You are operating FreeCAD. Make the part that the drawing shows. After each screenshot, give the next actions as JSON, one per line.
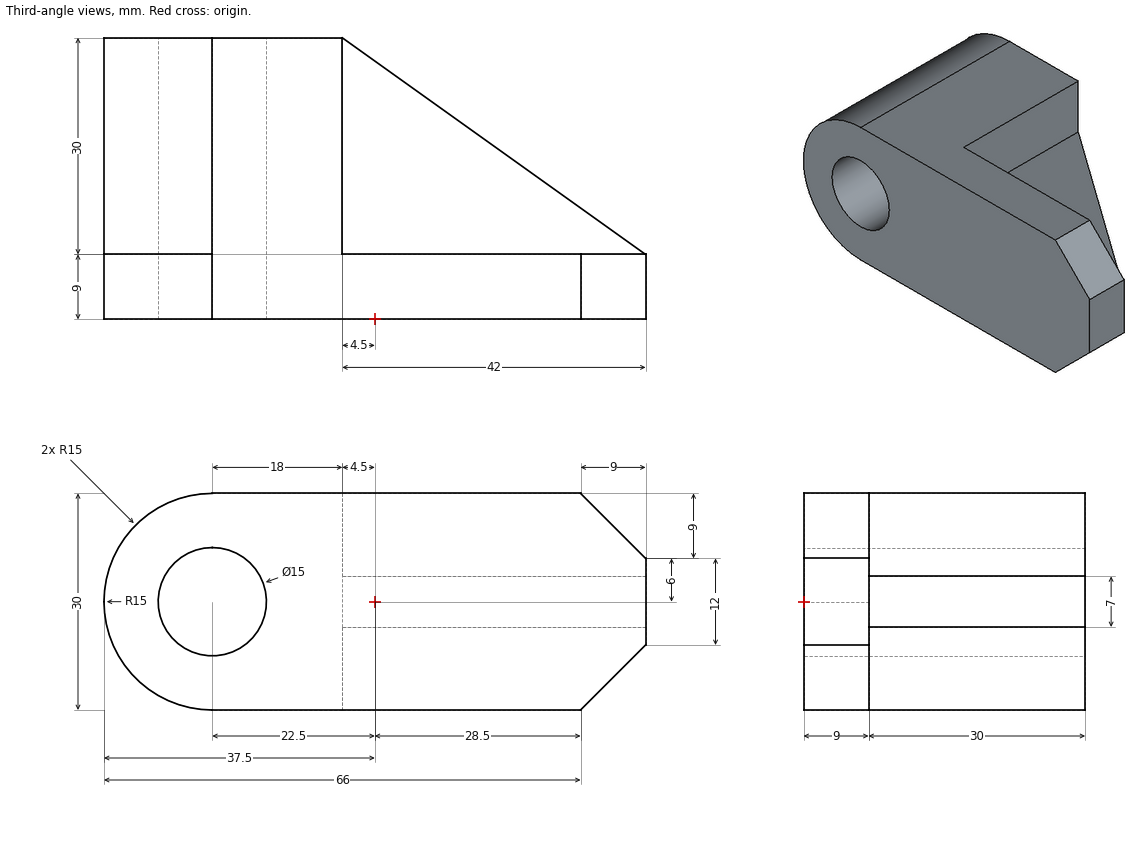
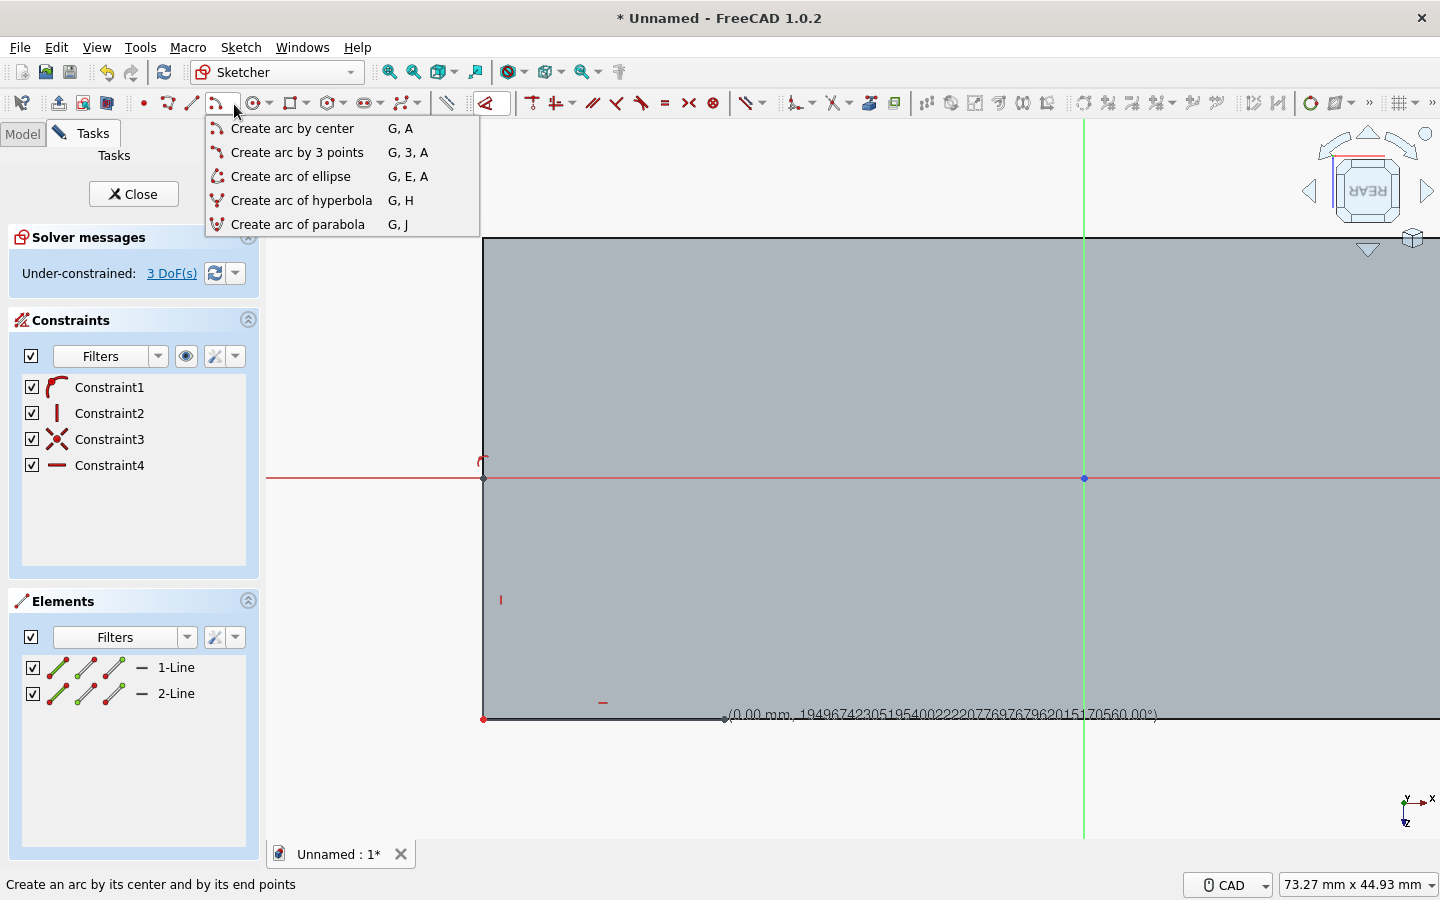
{"action": "left_click", "coordinate": [342, 152]}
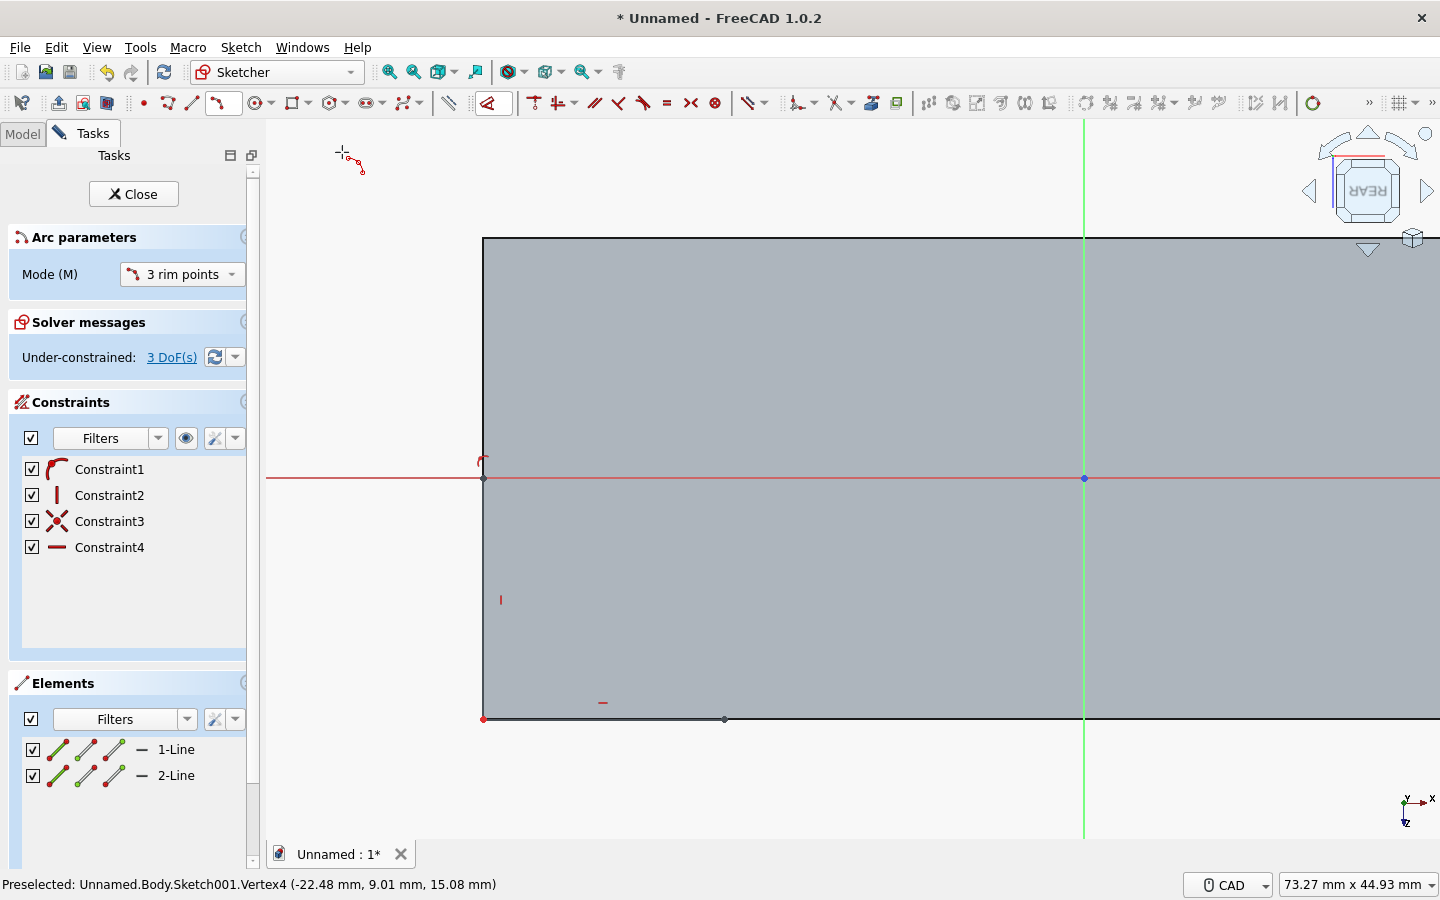
{"action": "left_click", "coordinate": [724, 720]}
{"action": "left_click", "coordinate": [483, 478]}
{"action": "left_click", "coordinate": [554, 648]}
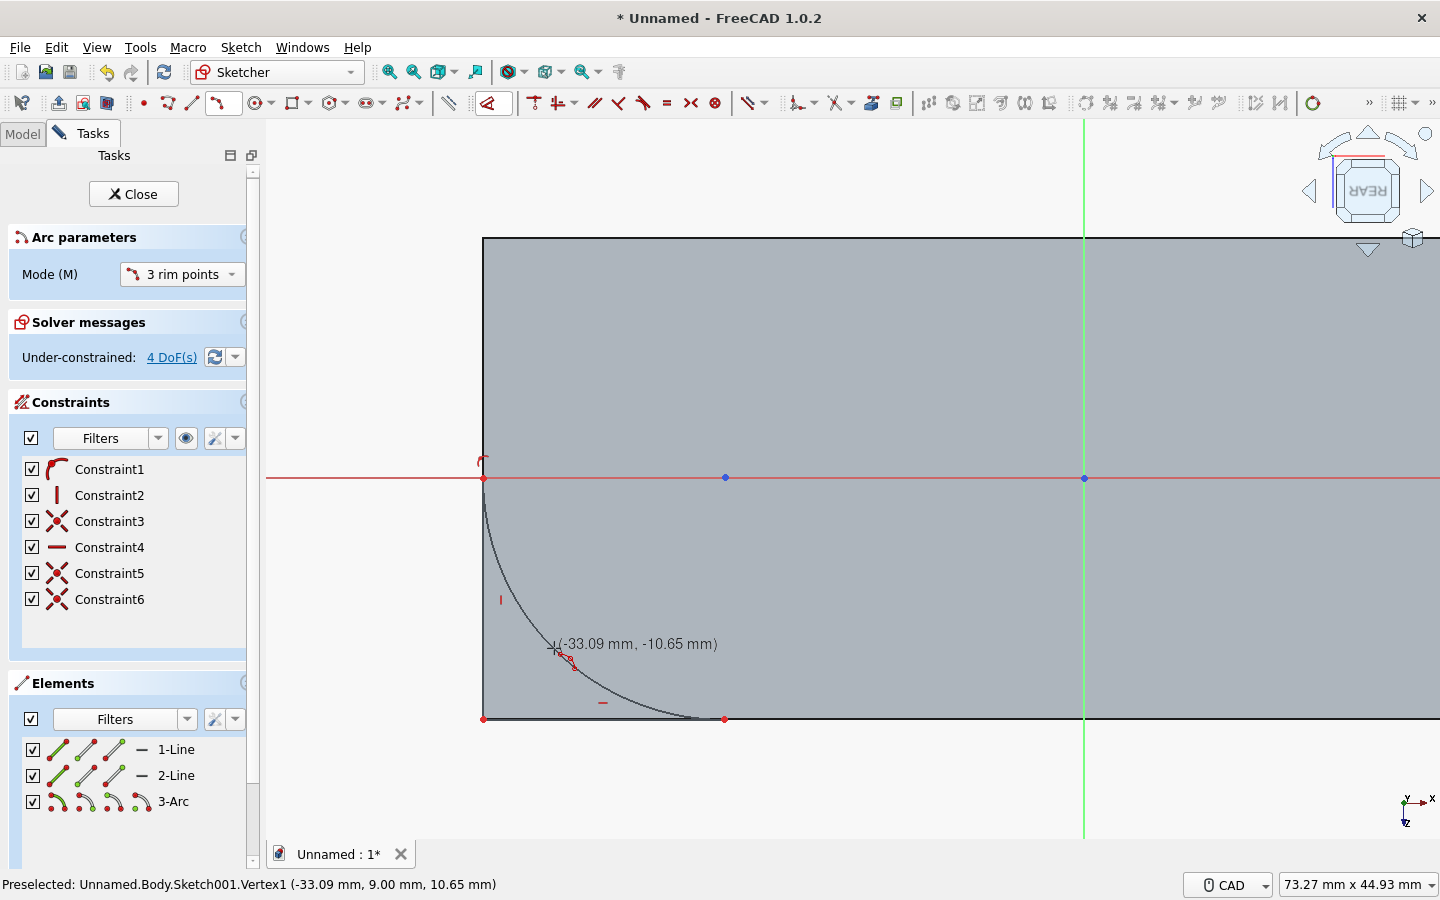
{"action": "key", "text": "g m"}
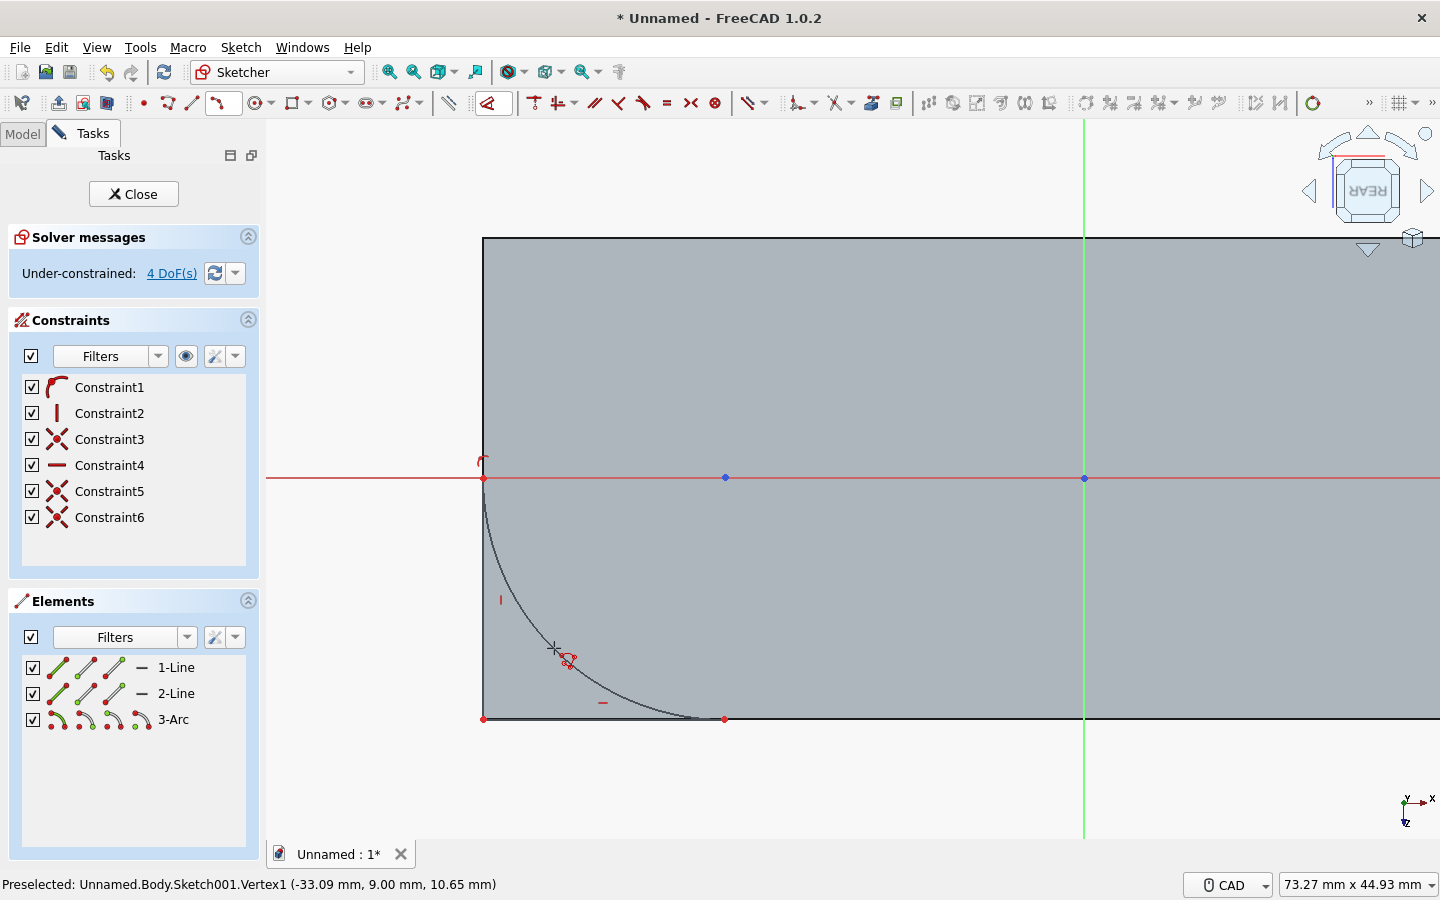
{"action": "left_click", "coordinate": [724, 238]}
{"action": "left_click", "coordinate": [483, 238]}
{"action": "left_click", "coordinate": [483, 478]}
{"action": "right_click", "coordinate": [483, 238]}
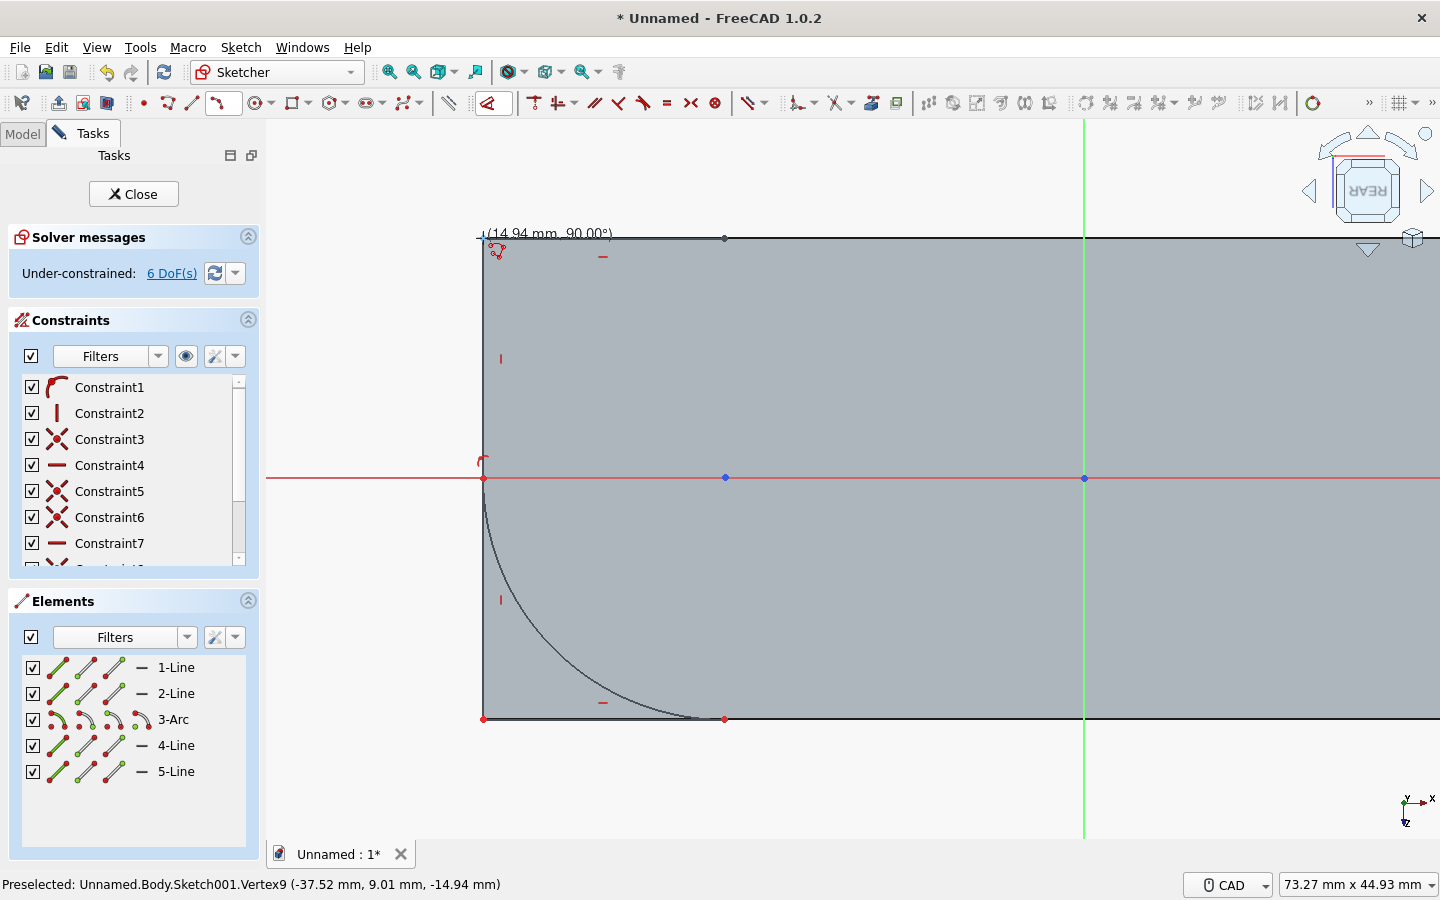
{"action": "left_click", "coordinate": [218, 104]}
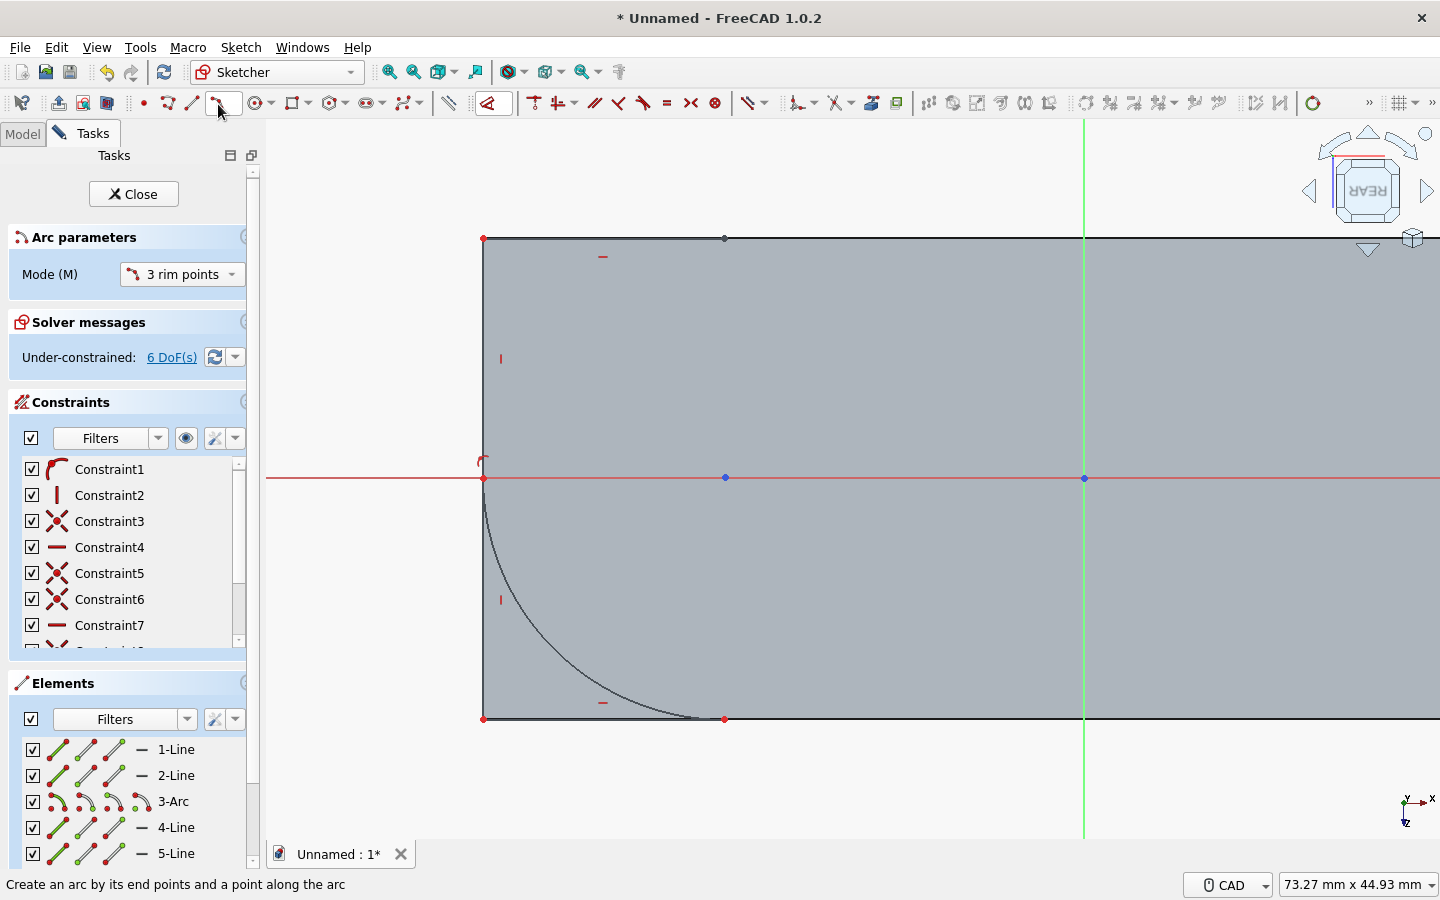
{"action": "left_click", "coordinate": [483, 478]}
{"action": "left_click", "coordinate": [724, 239]}
{"action": "left_click", "coordinate": [554, 308]}
{"action": "key", "text": "Escape"}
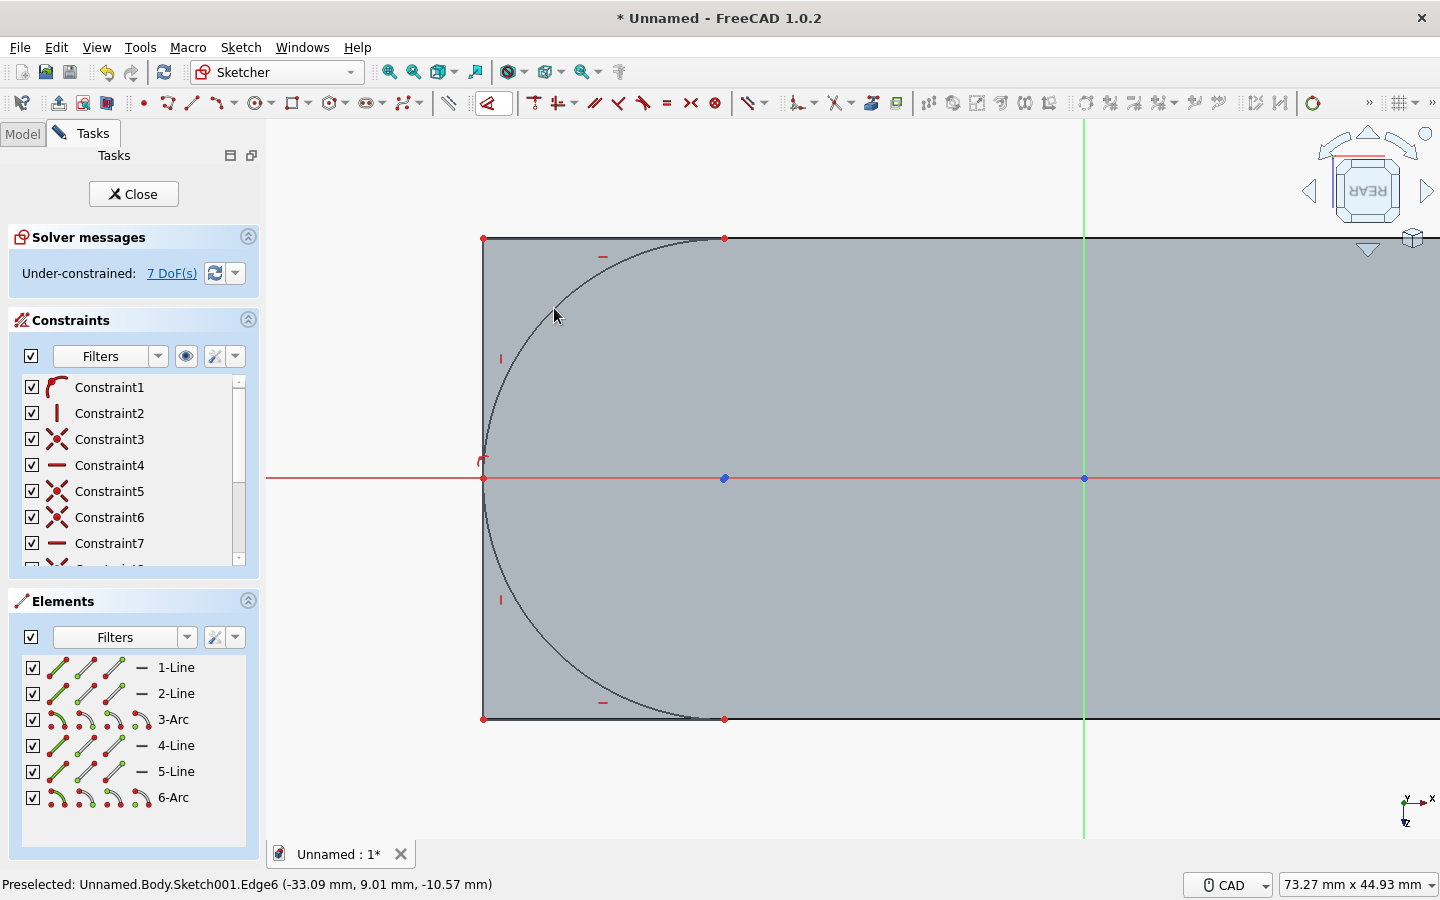
{"action": "scroll", "coordinate": [483, 551], "scroll_direction": "up", "scroll_amount": 2}